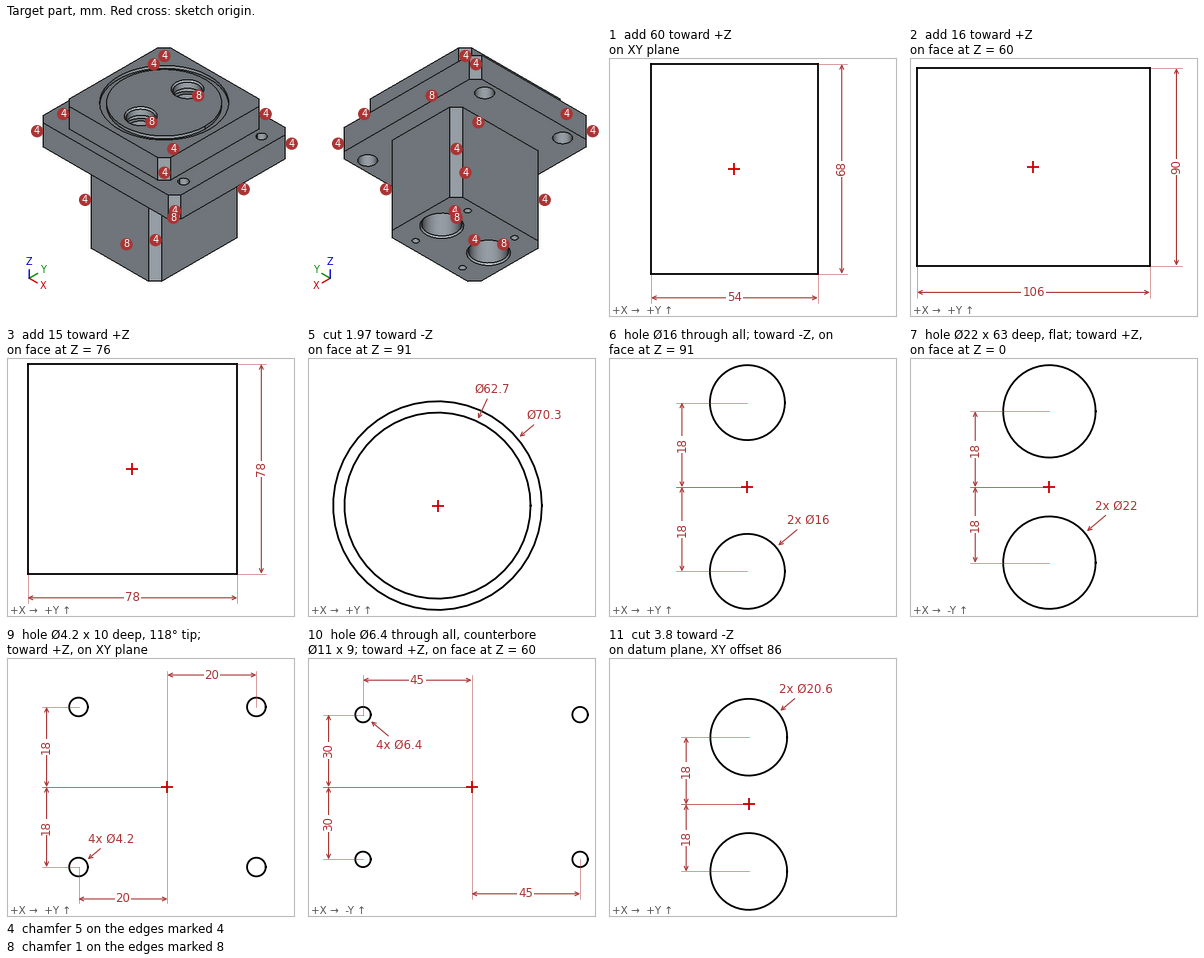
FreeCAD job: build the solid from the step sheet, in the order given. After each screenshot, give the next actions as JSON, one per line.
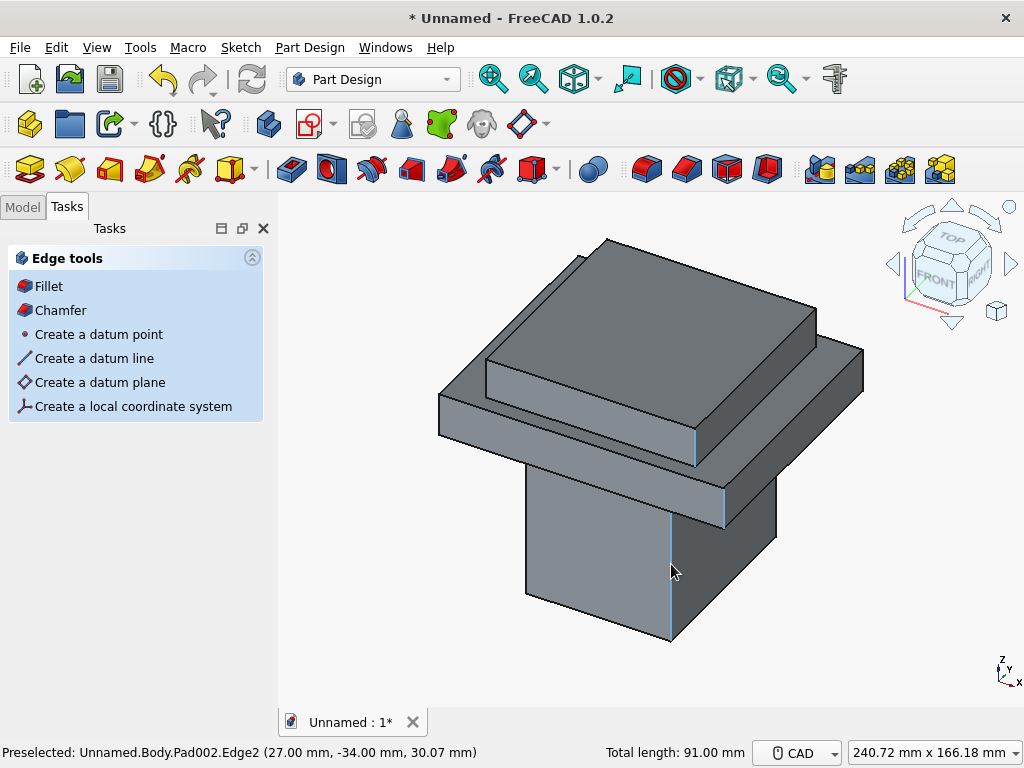
{"action": "key", "text": "0"}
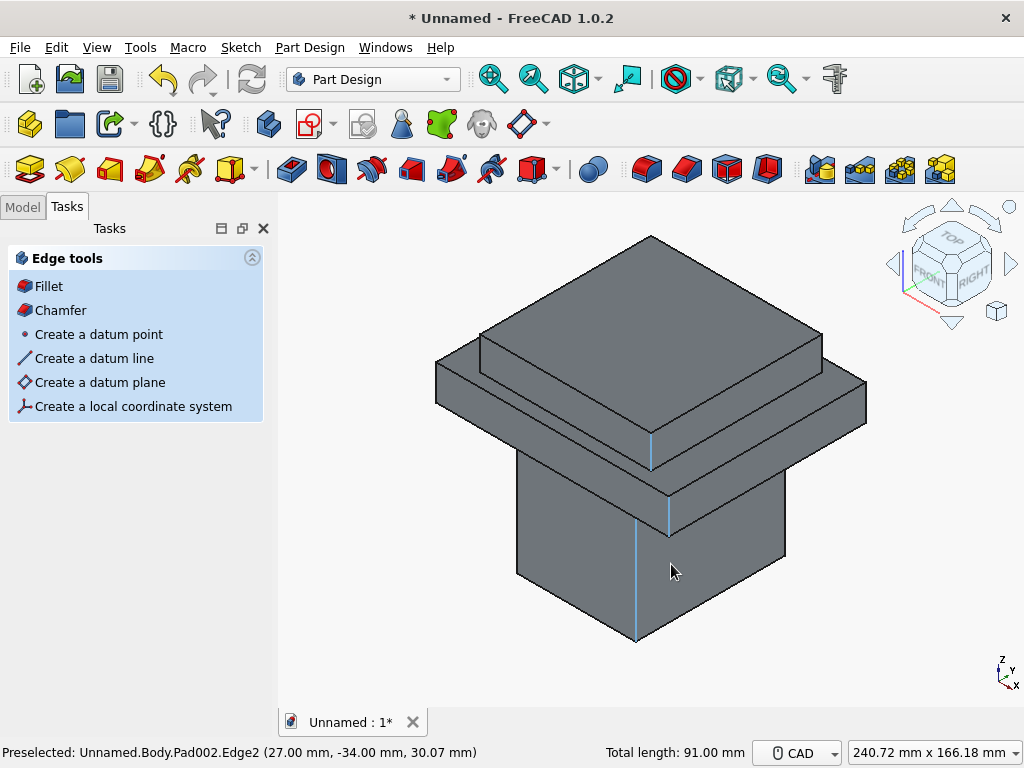
{"action": "key", "text": "2"}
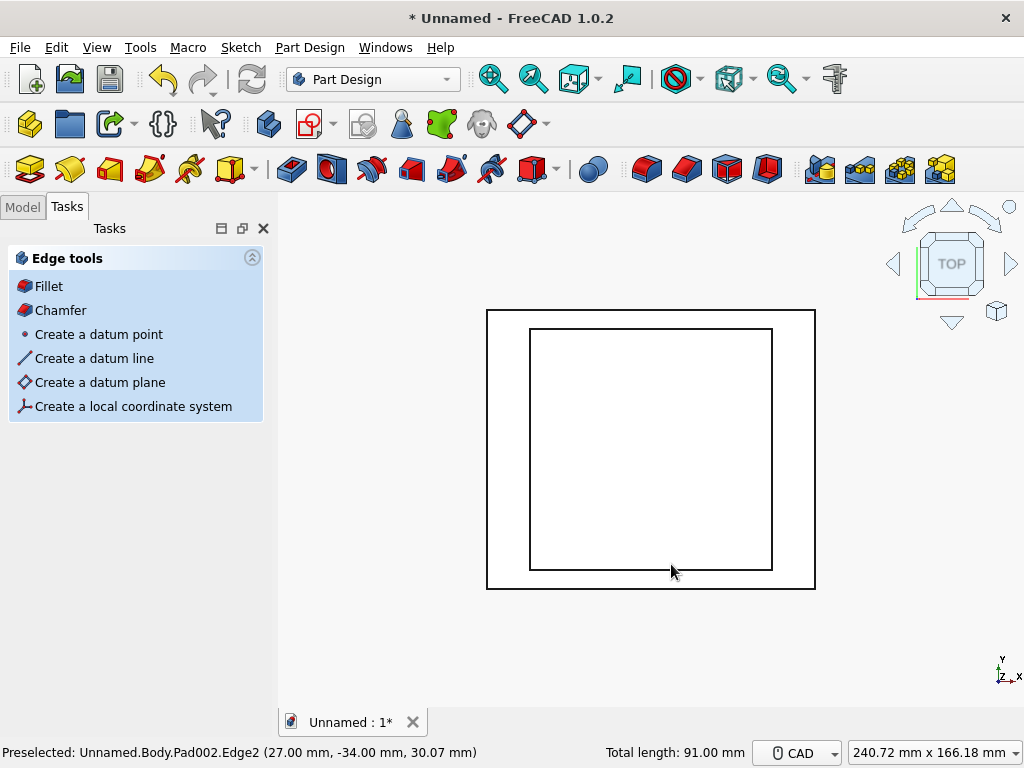
{"action": "key", "text": "1"}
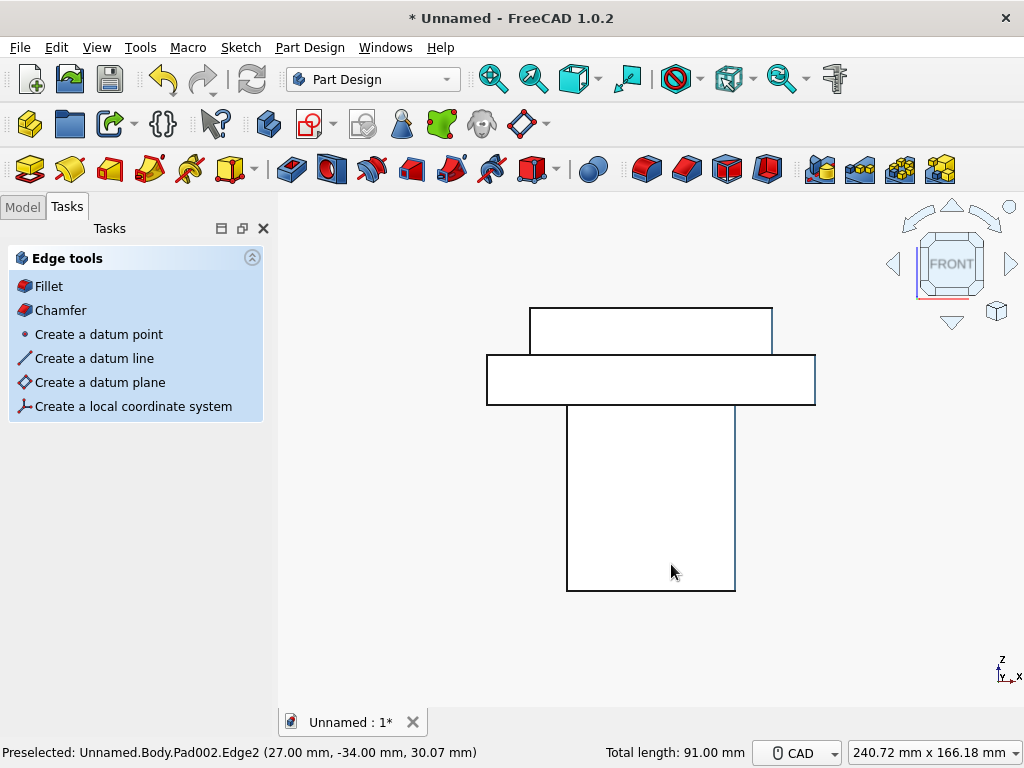
{"action": "left_click", "coordinate": [487, 379], "text": "ctrl"}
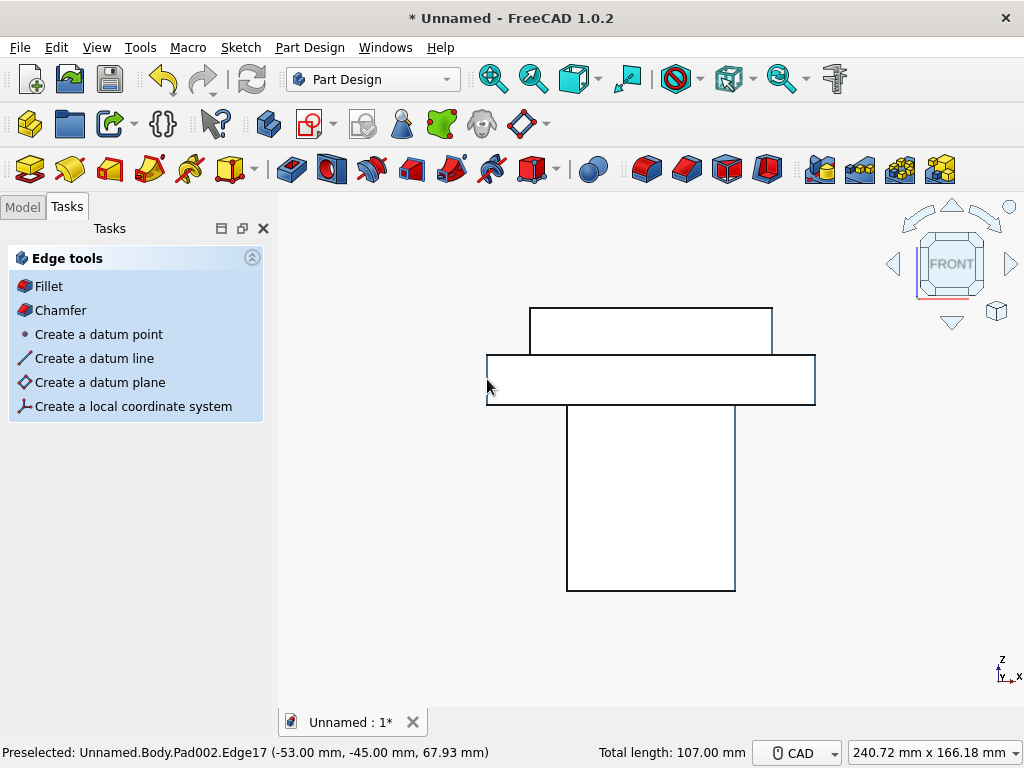
{"action": "left_click", "coordinate": [530, 331], "text": "ctrl"}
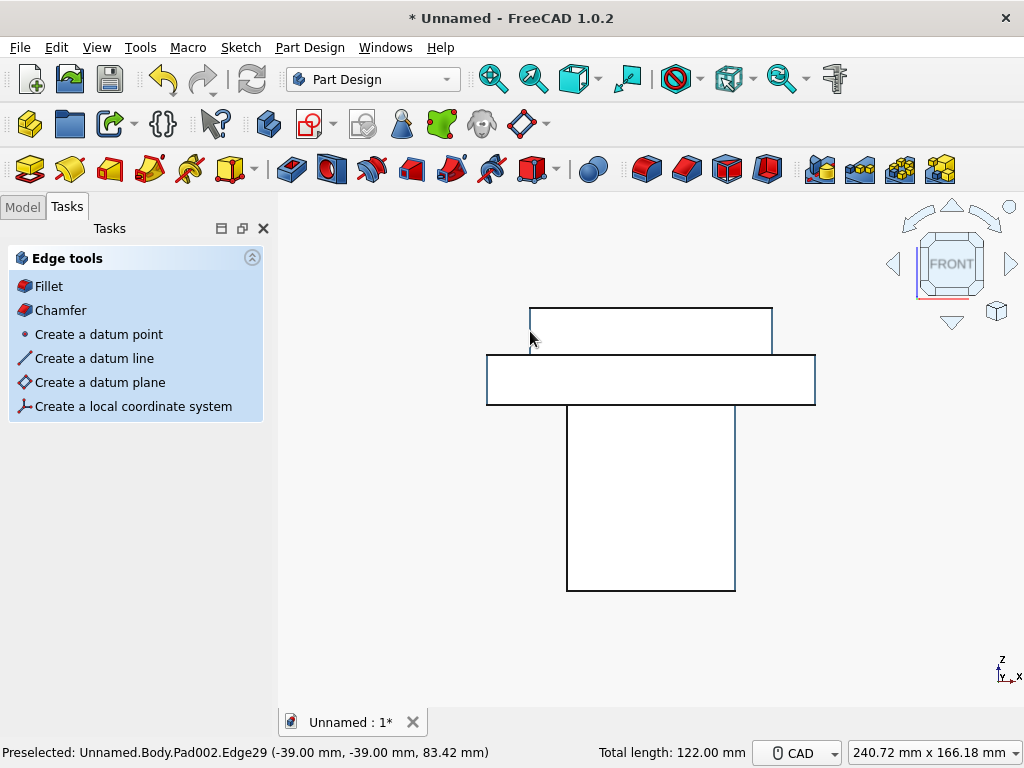
{"action": "left_click", "coordinate": [567, 497], "text": "ctrl"}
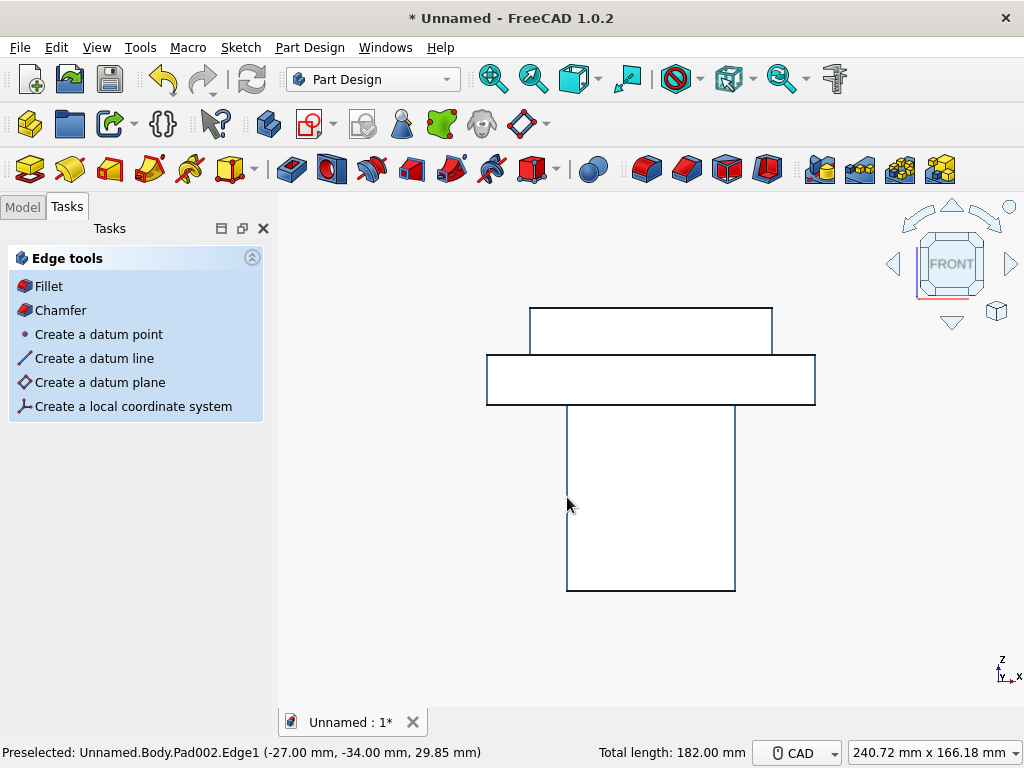
{"action": "key", "text": "3"}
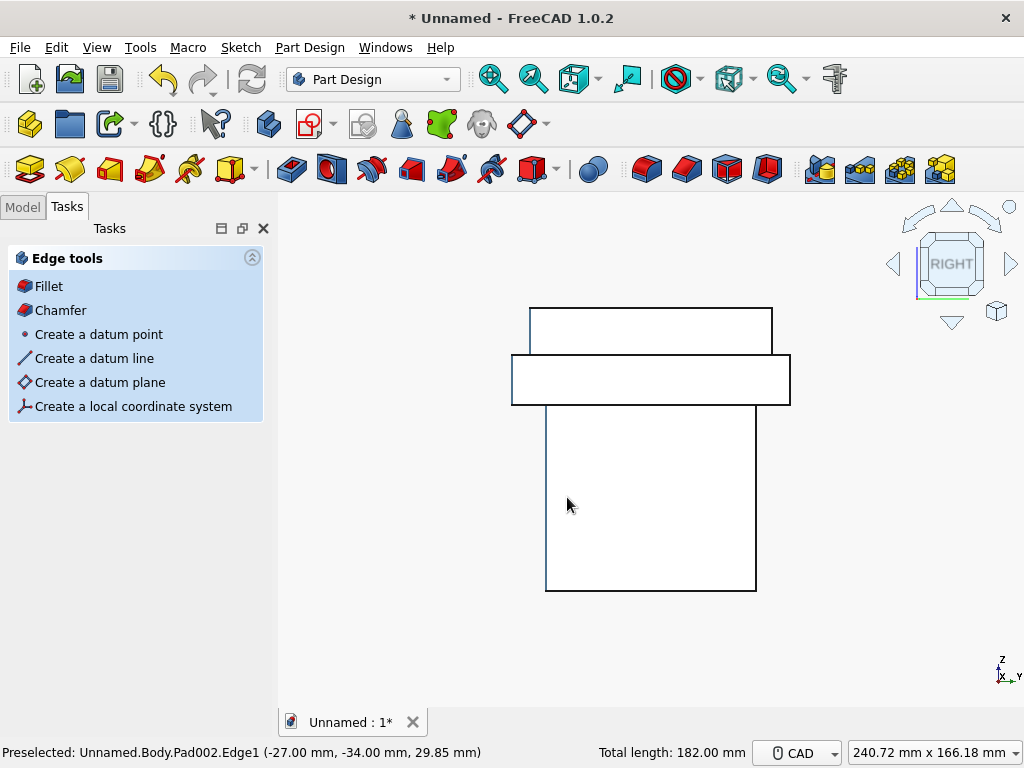
{"action": "left_click", "coordinate": [790, 379], "text": "ctrl"}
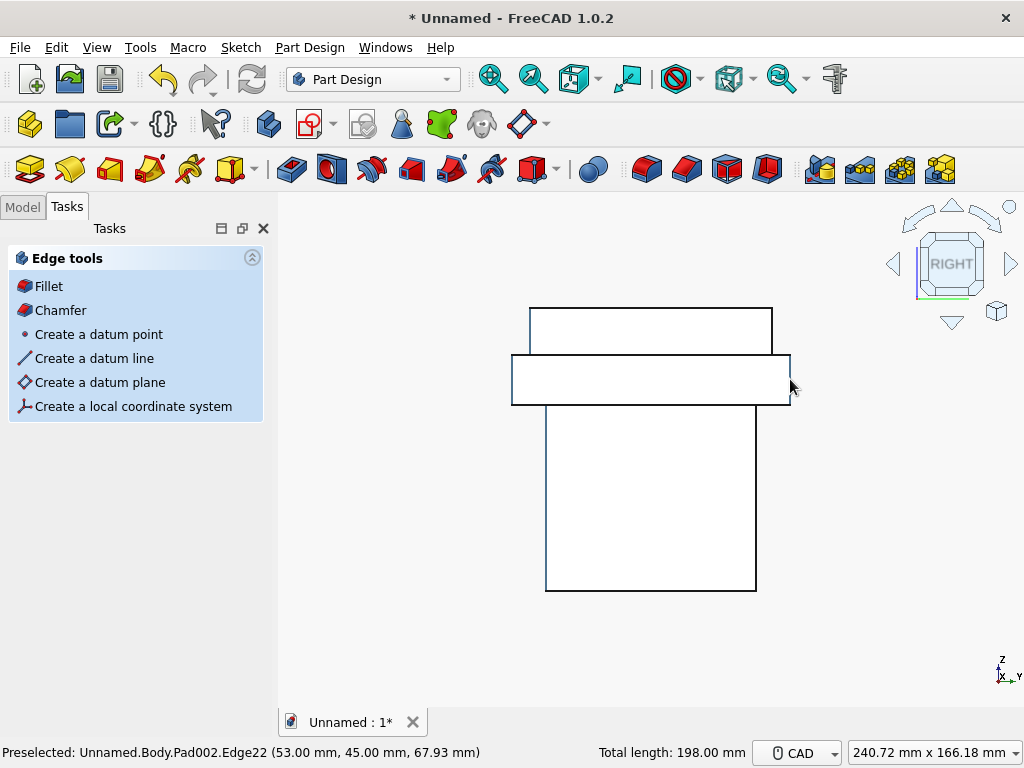
{"action": "left_click", "coordinate": [772, 331], "text": "ctrl"}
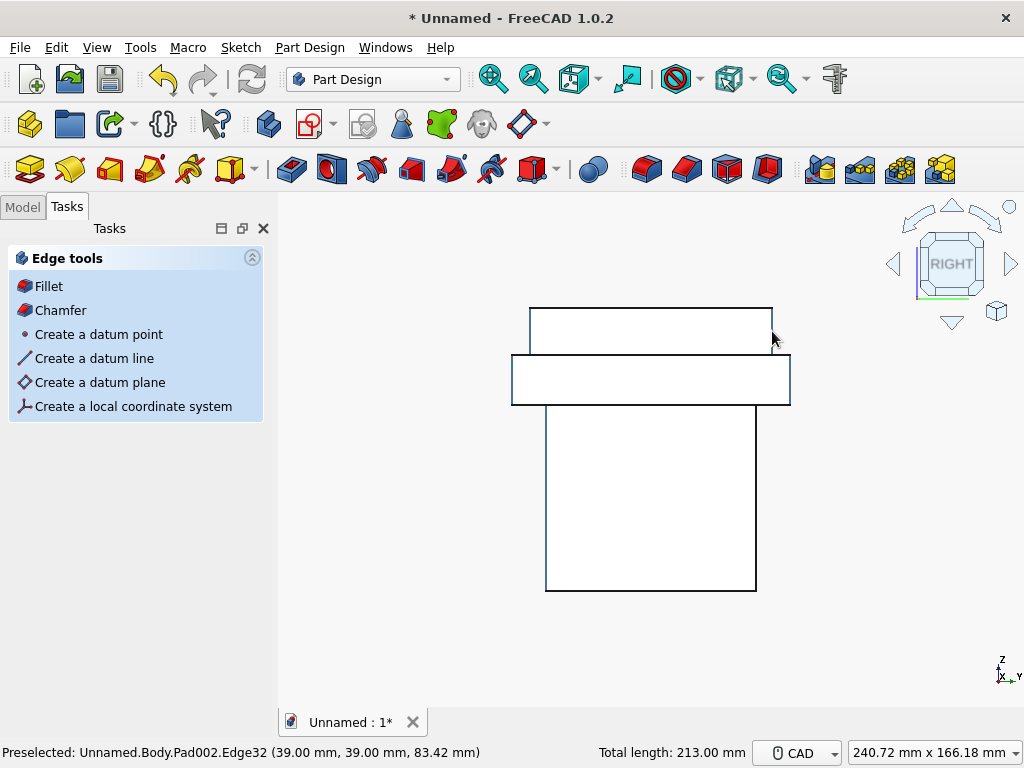
{"action": "left_click", "coordinate": [756, 497], "text": "ctrl"}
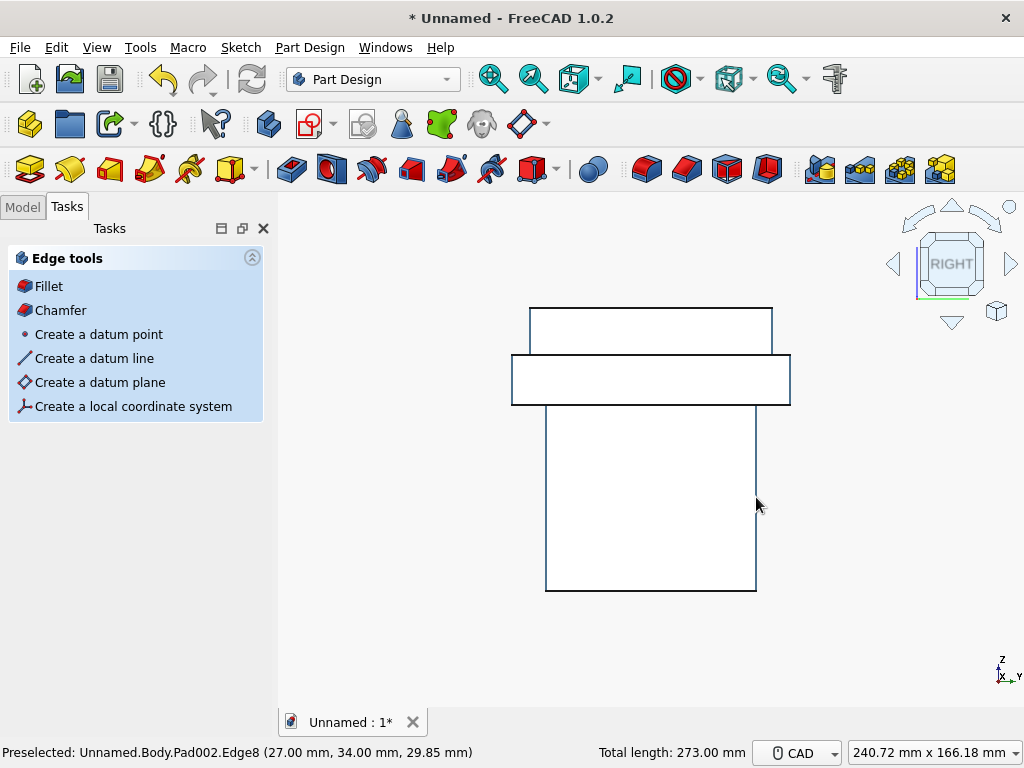
{"action": "key", "text": "5"}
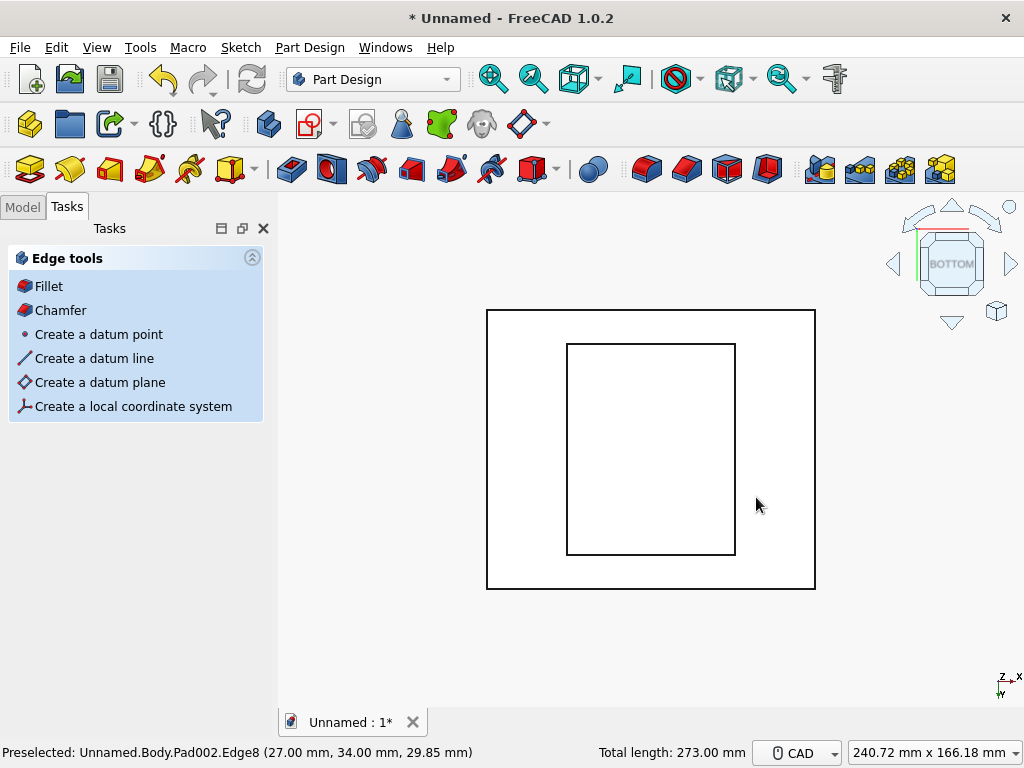
{"action": "key", "text": "4"}